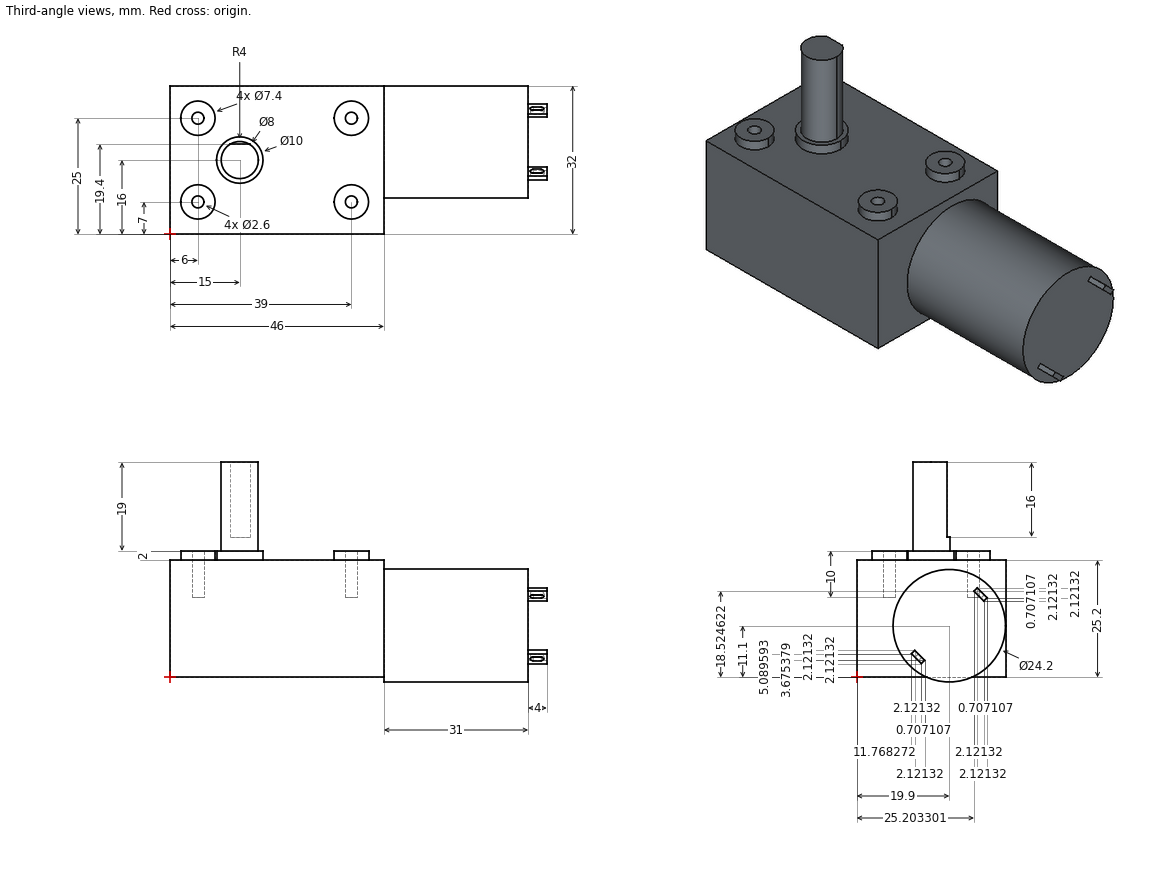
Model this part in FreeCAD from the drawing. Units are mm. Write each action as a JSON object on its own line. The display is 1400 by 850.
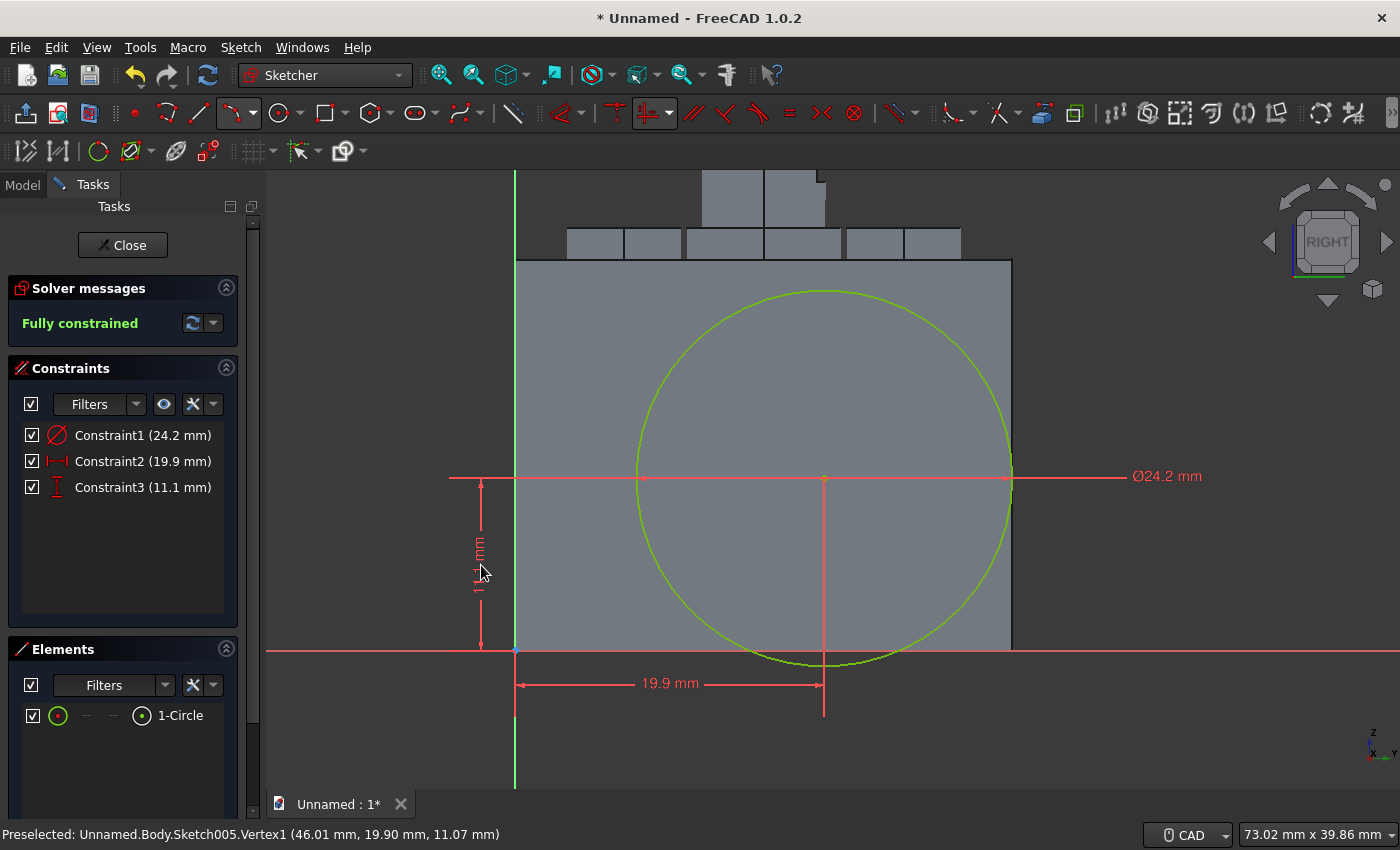
{"action": "left_click", "coordinate": [123, 245]}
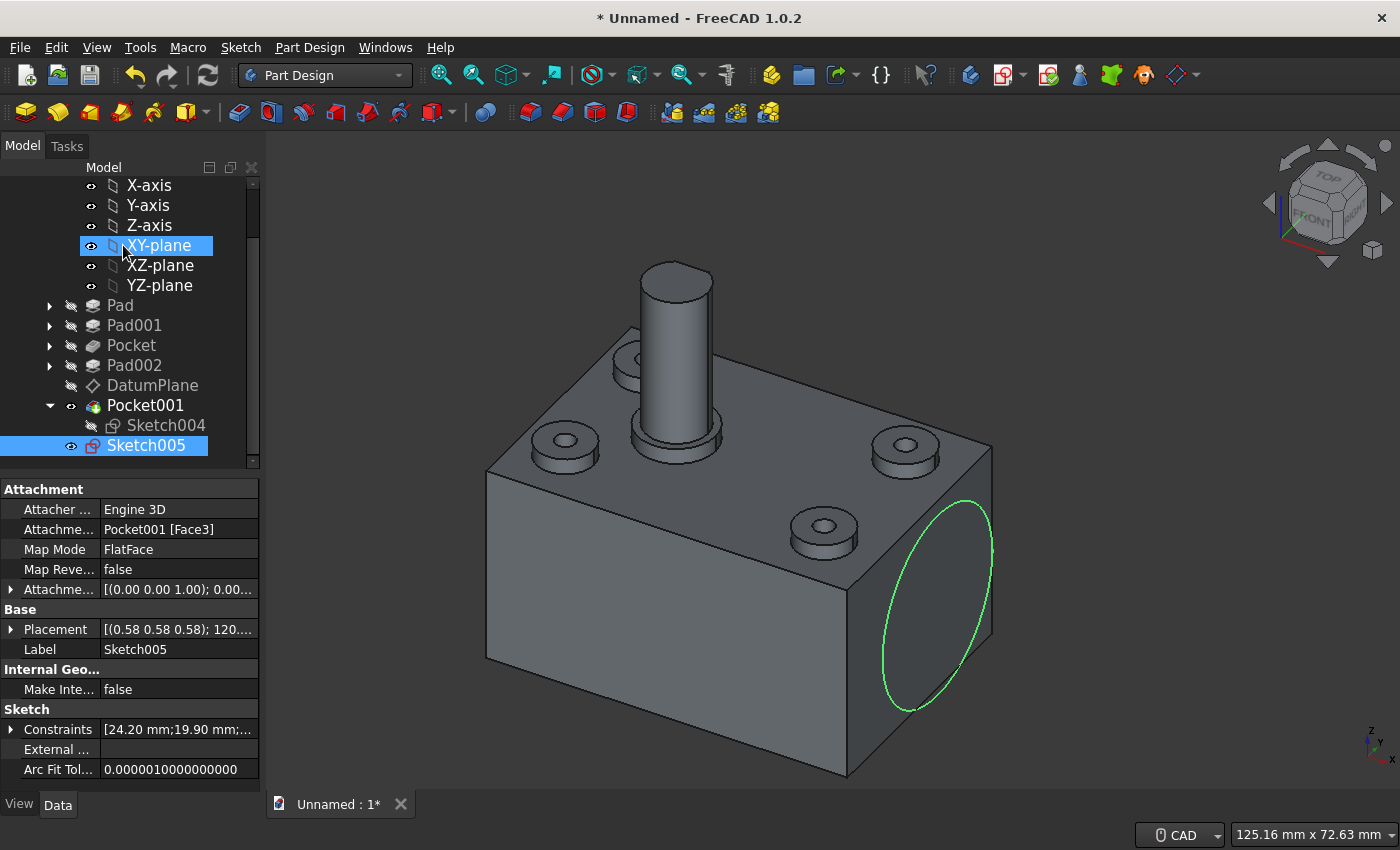
{"action": "left_click", "coordinate": [26, 112]}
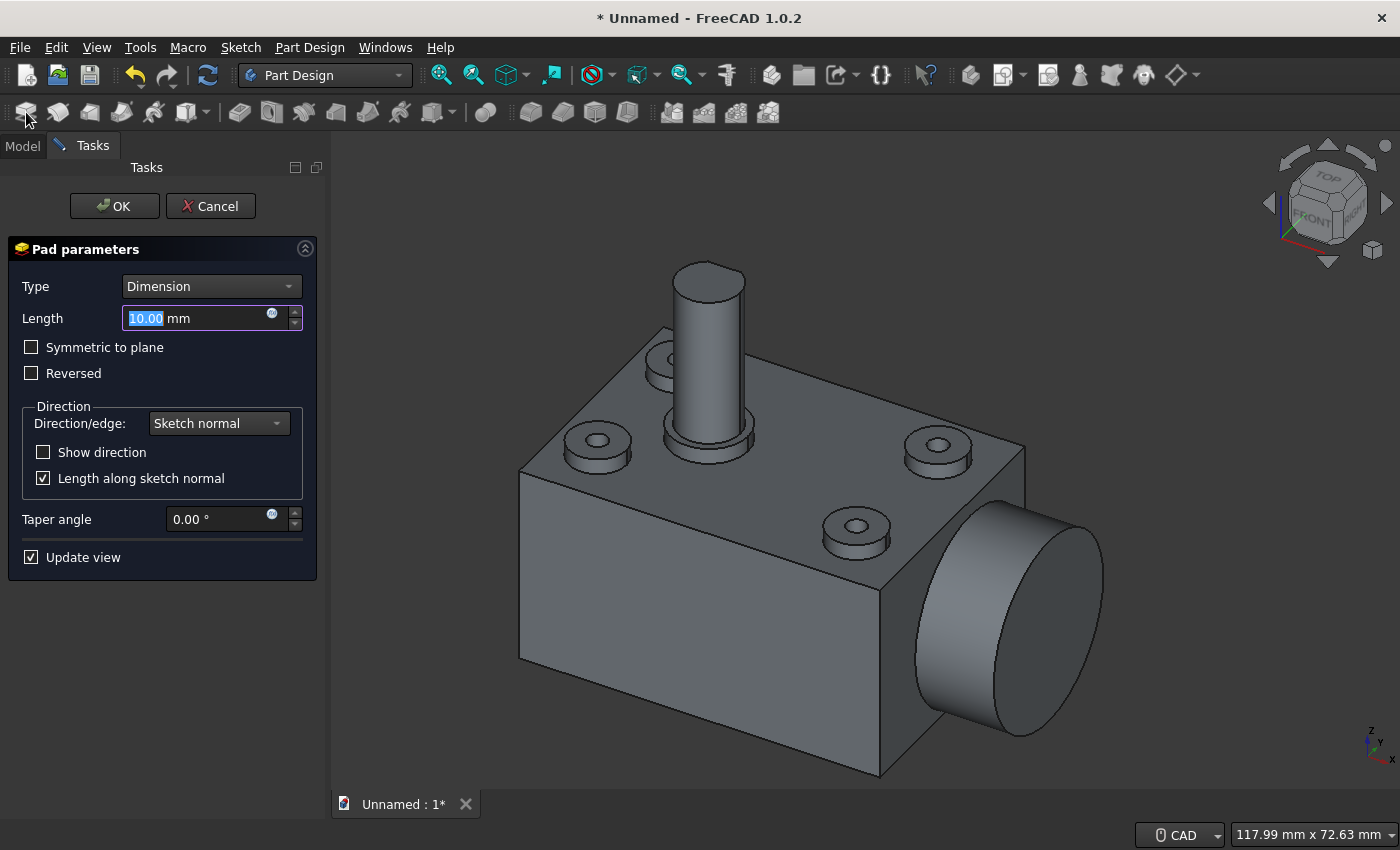
{"action": "type", "text": "31"}
{"action": "key", "text": "Tab"}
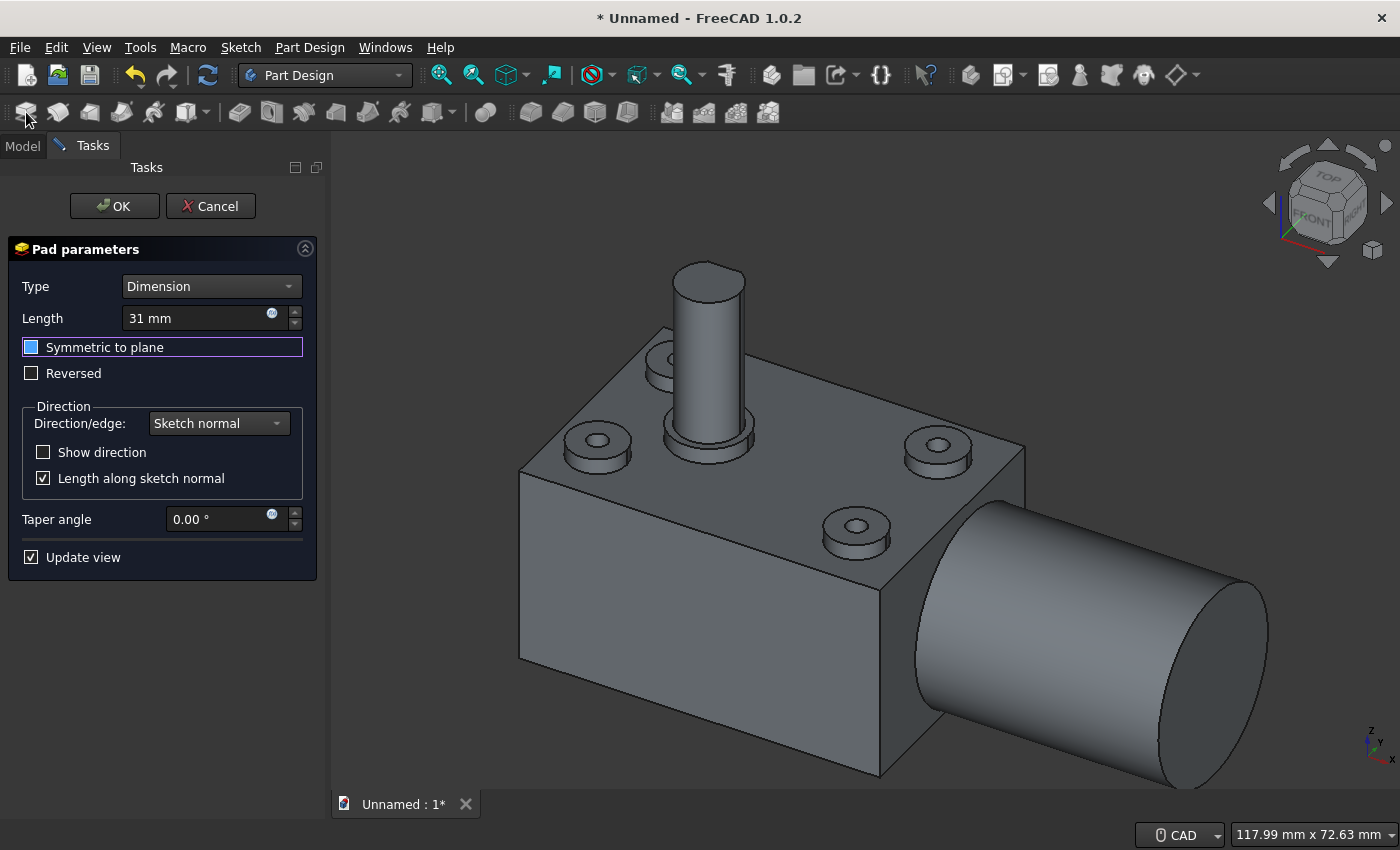
{"action": "left_click", "coordinate": [115, 206]}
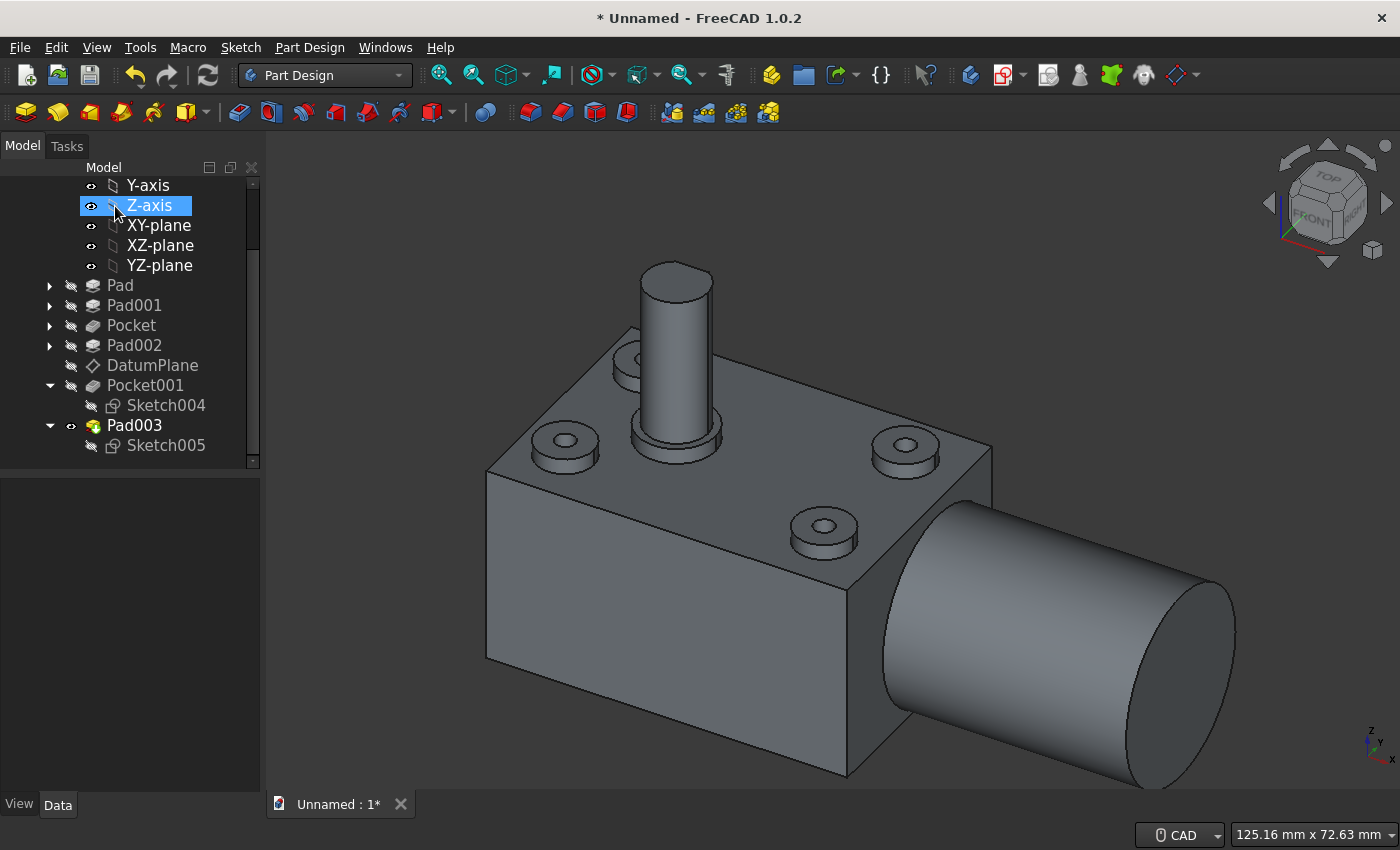
{"action": "left_click", "coordinate": [442, 76]}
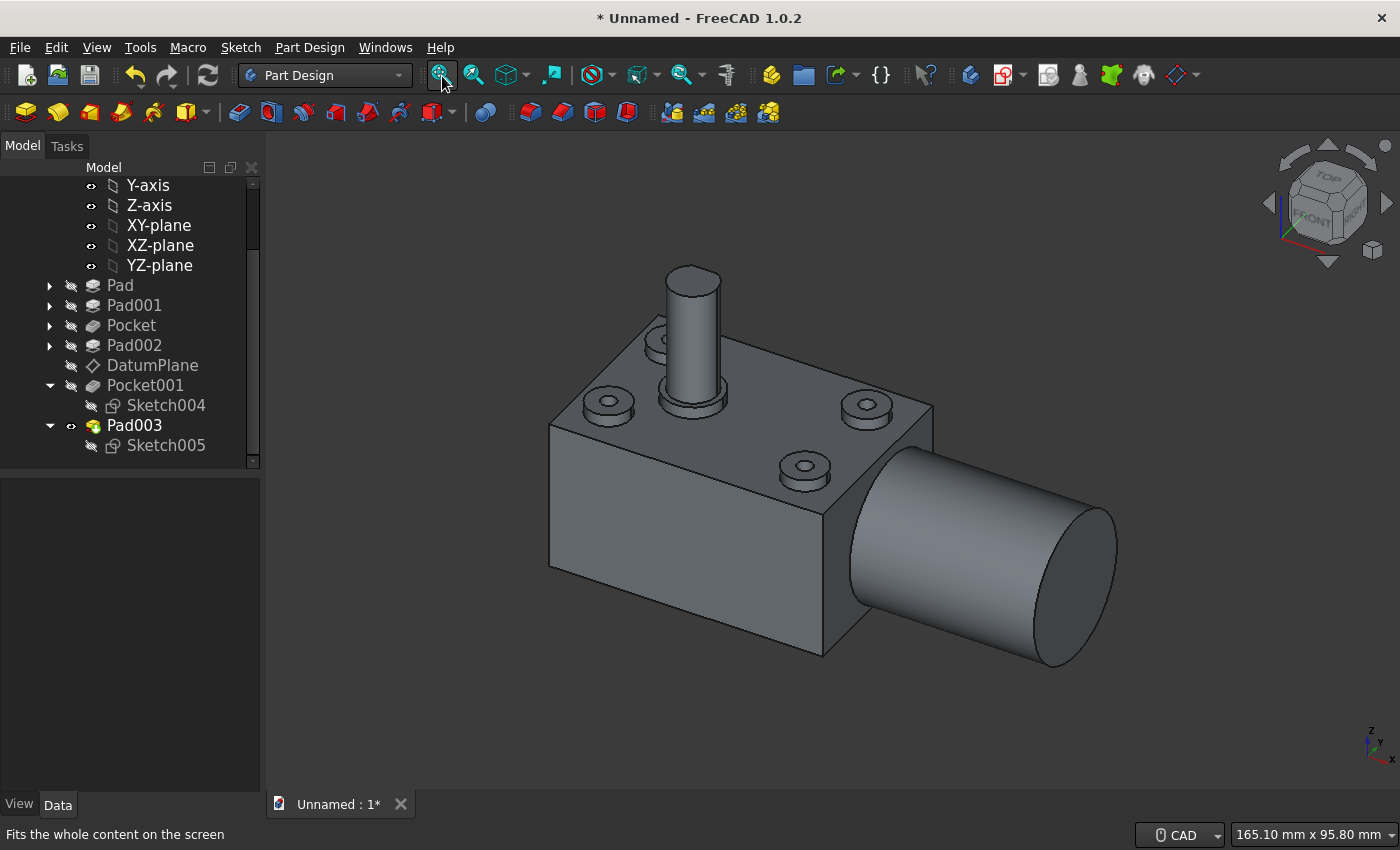
{"action": "left_click", "coordinate": [1075, 586]}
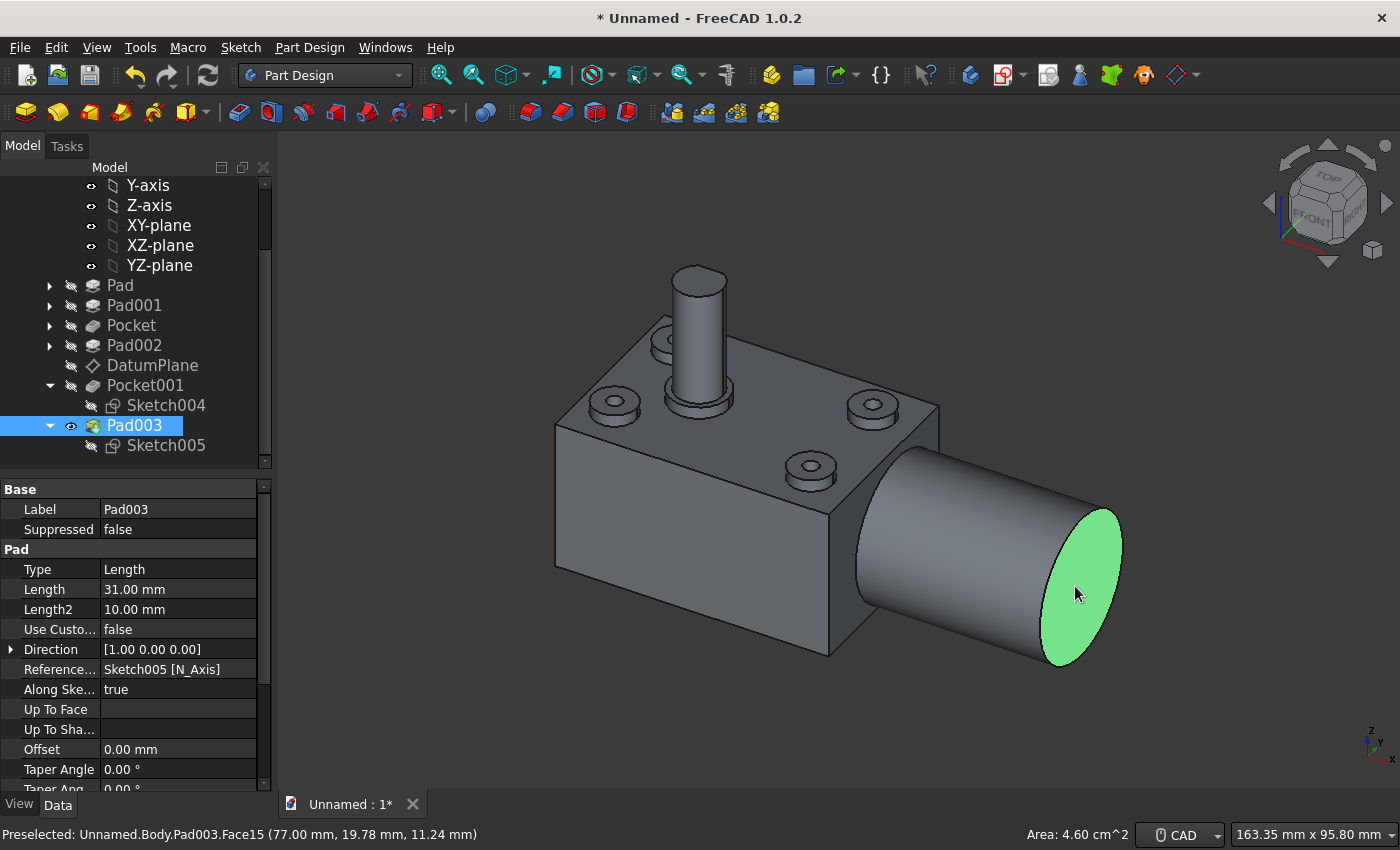
{"action": "left_click", "coordinate": [1004, 76]}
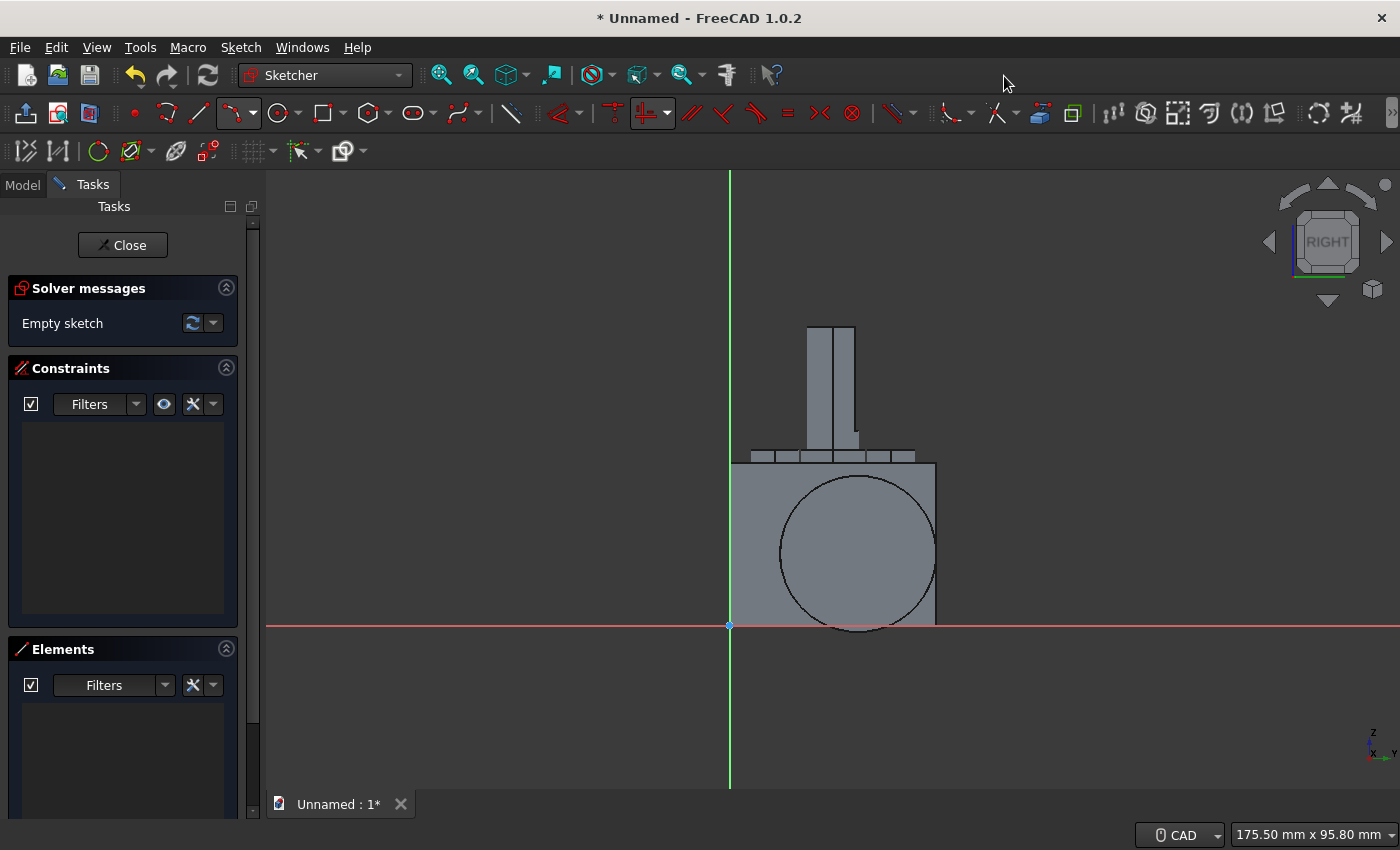
{"action": "scroll", "coordinate": [844, 600], "scroll_direction": "up", "scroll_amount": 6}